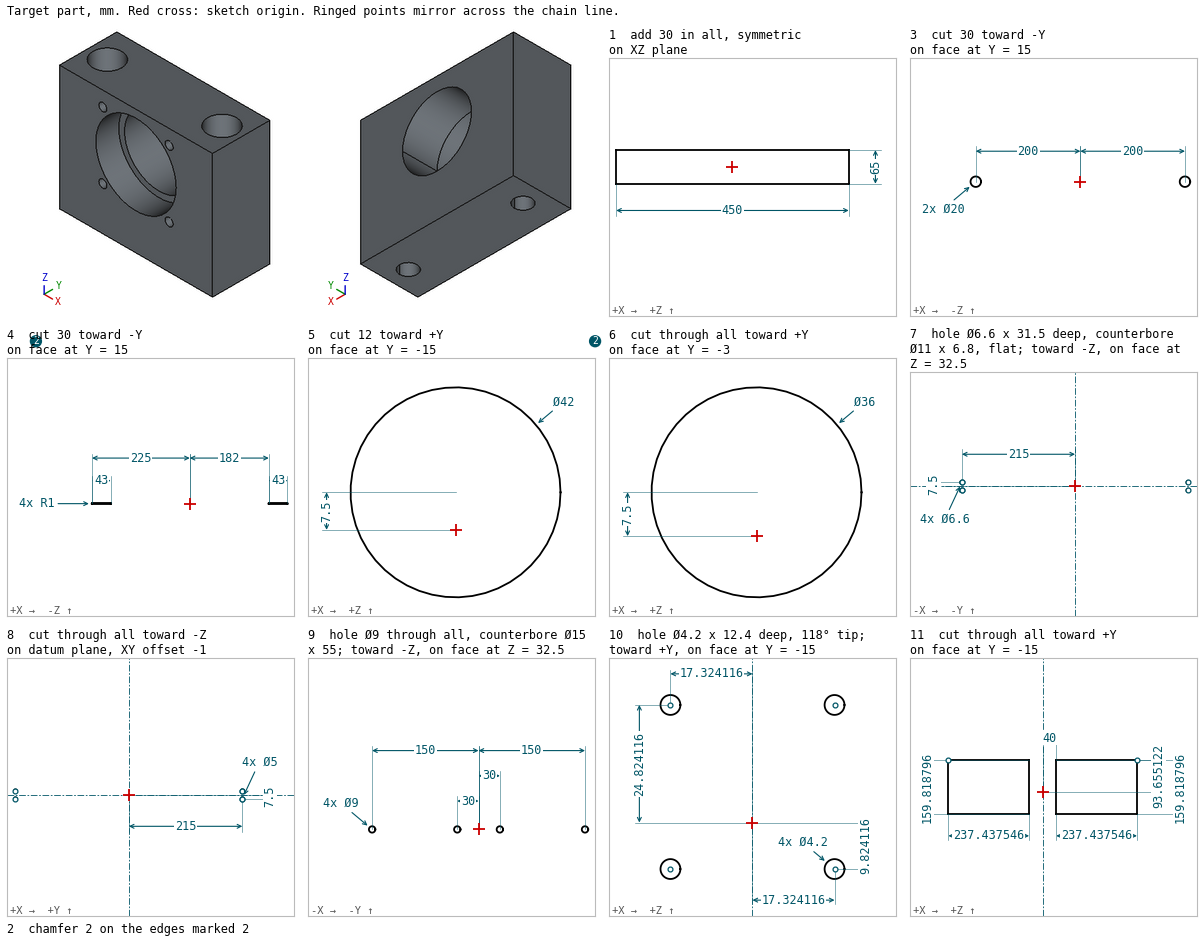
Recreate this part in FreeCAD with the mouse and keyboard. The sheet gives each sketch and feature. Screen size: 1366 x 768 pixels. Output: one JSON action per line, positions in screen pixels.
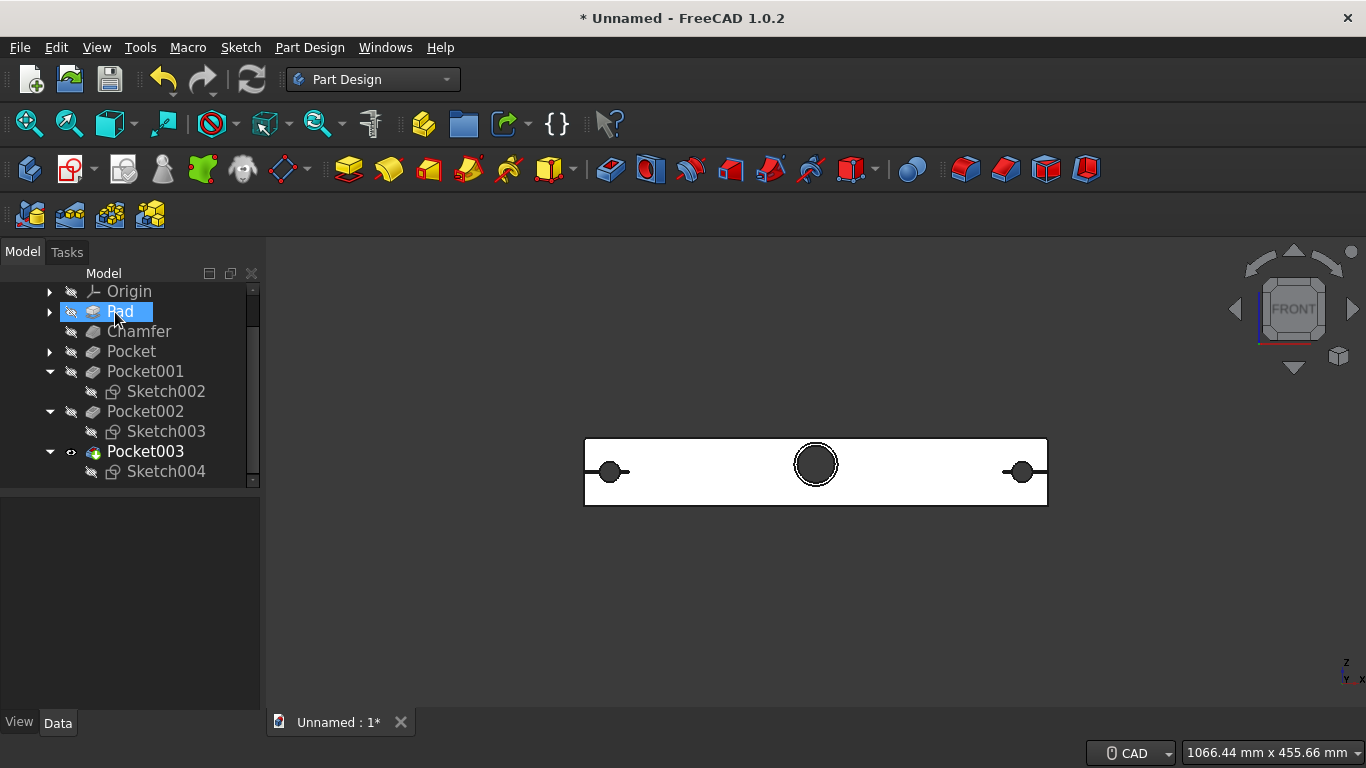
{"action": "key", "text": "0"}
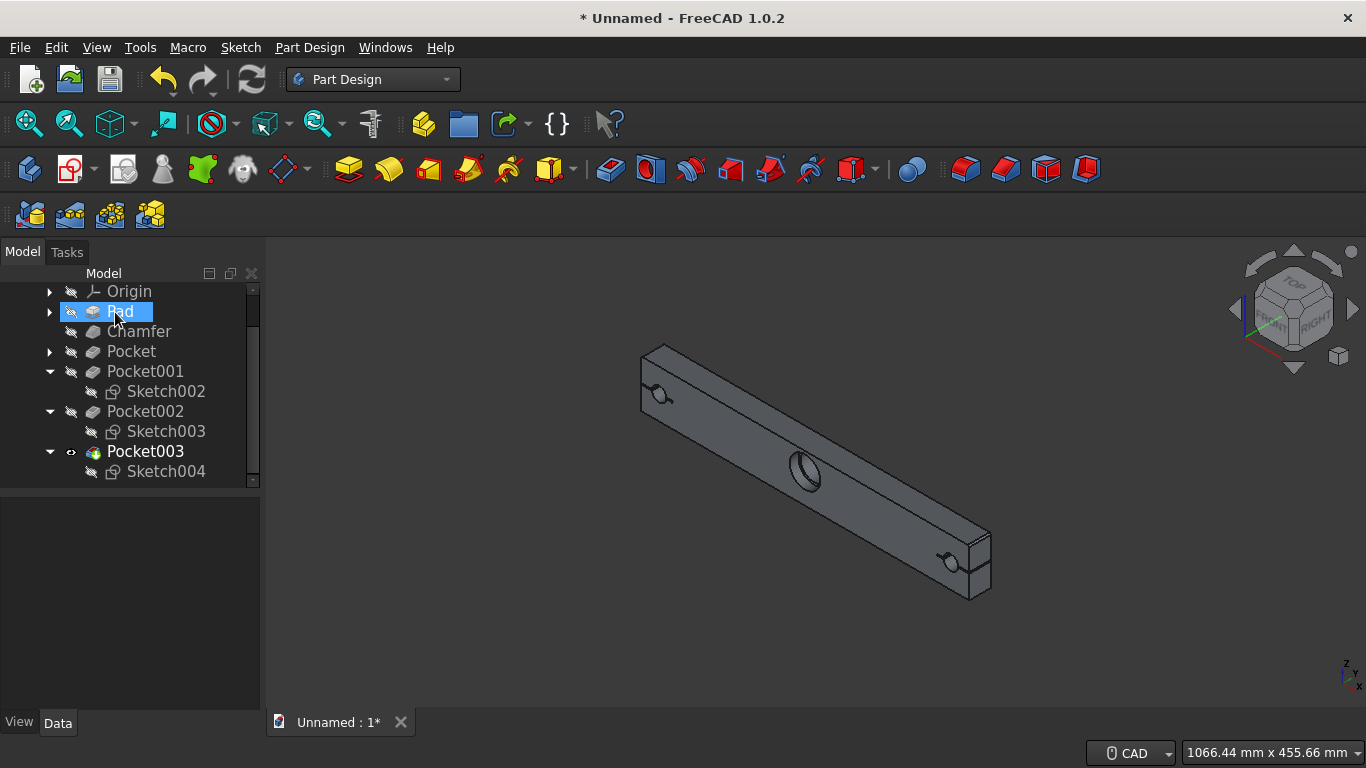
{"action": "left_click", "coordinate": [955, 524]}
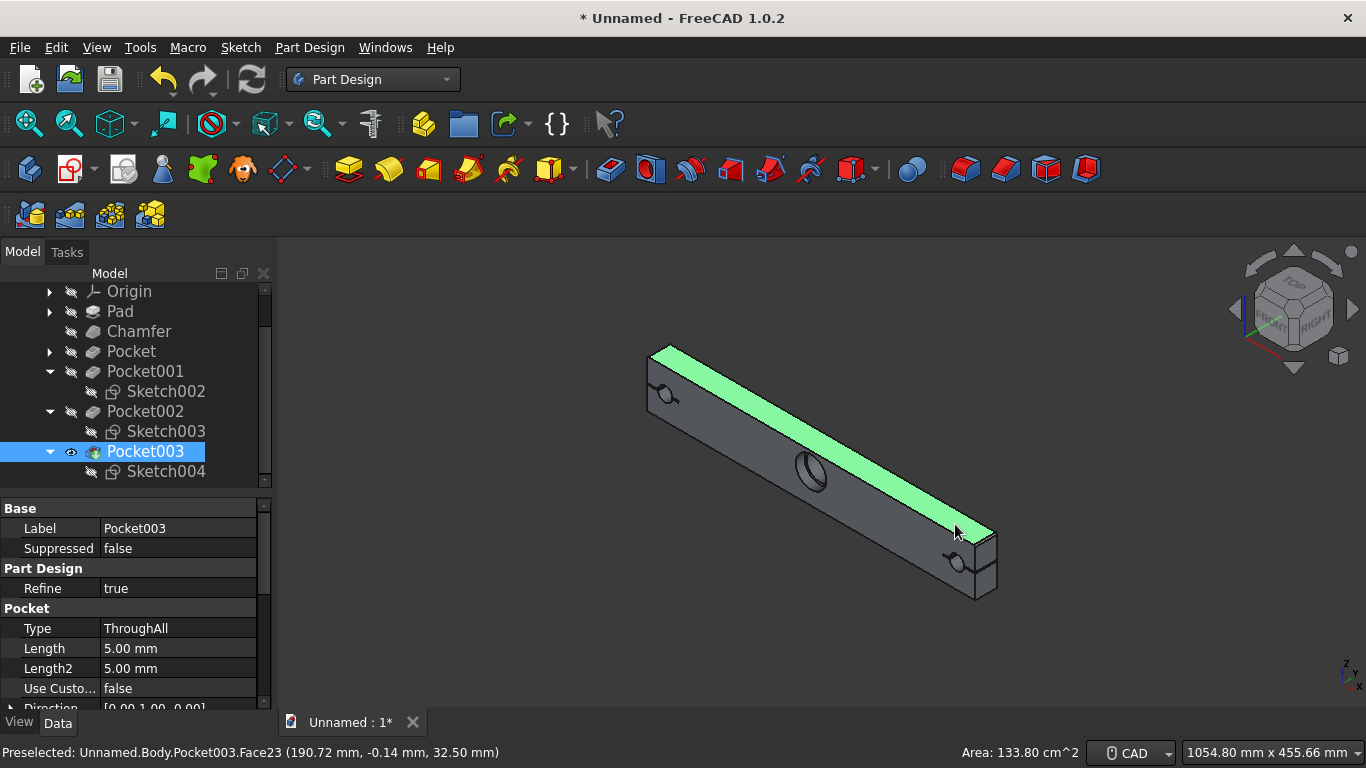
{"action": "left_click", "coordinate": [70, 170]}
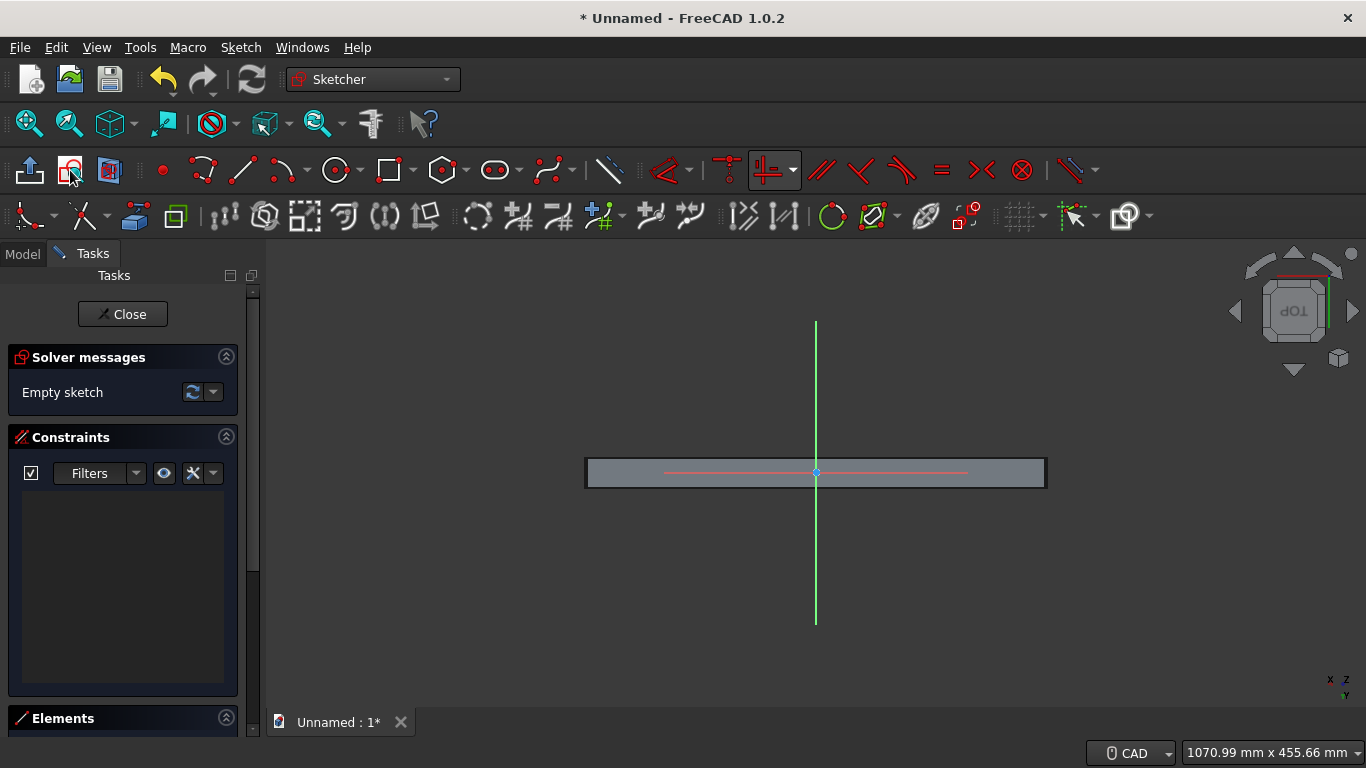
{"action": "scroll", "coordinate": [955, 473], "scroll_direction": "up", "scroll_amount": 2}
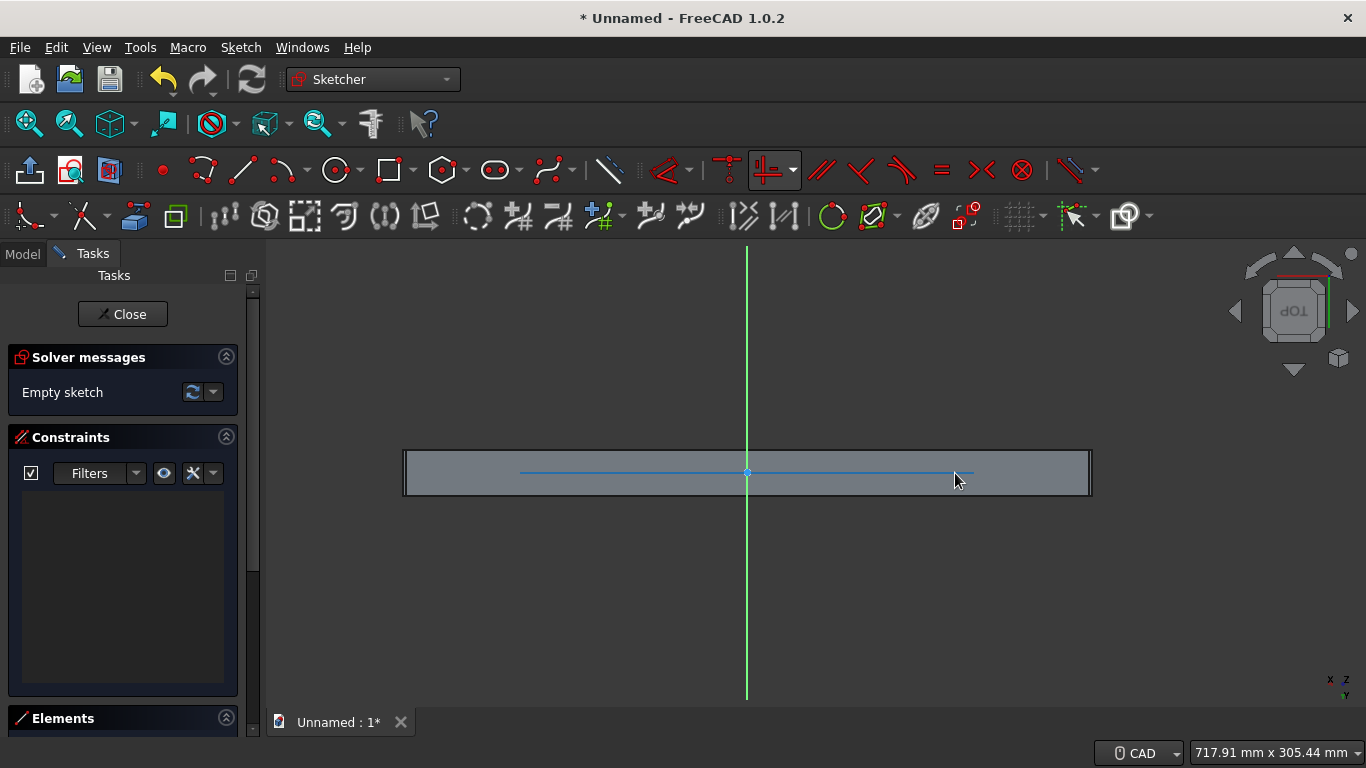
{"action": "key", "text": "g c"}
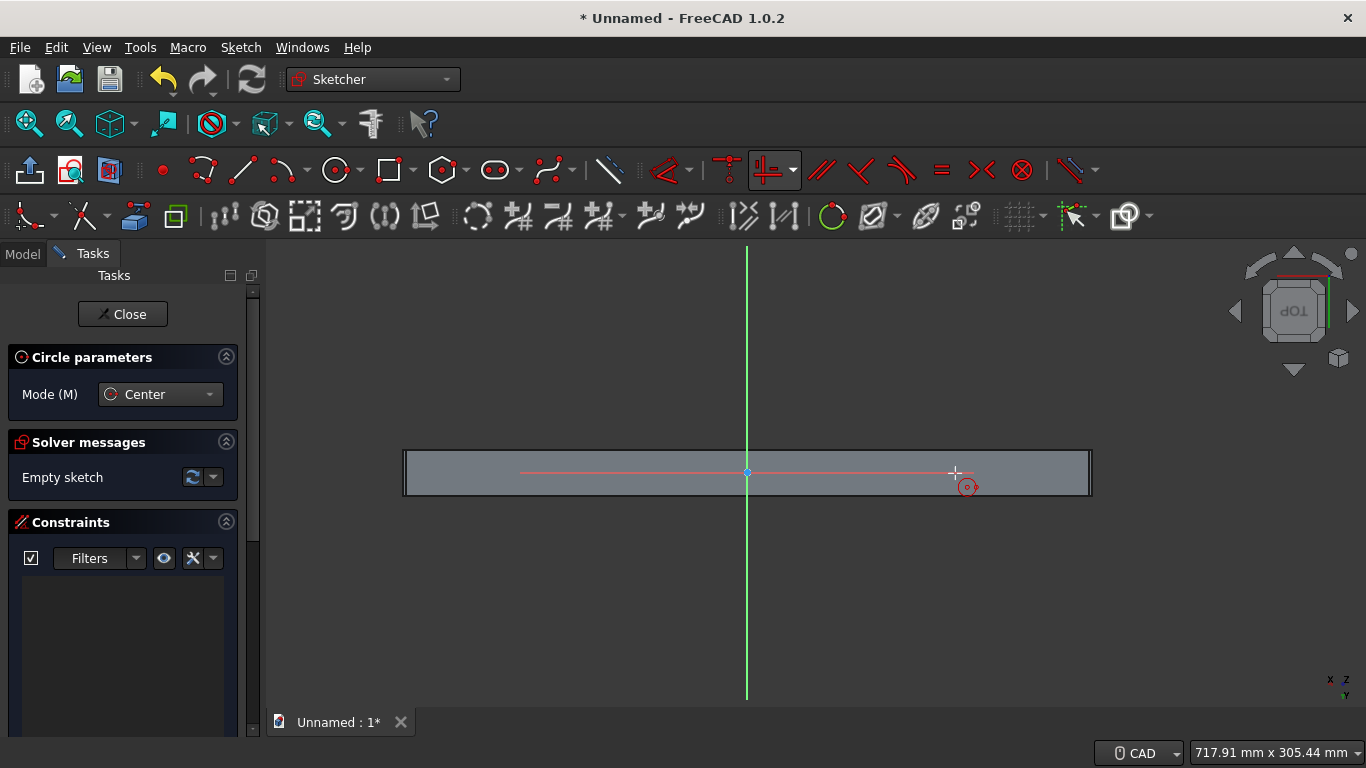
{"action": "scroll", "coordinate": [418, 461], "scroll_direction": "up", "scroll_amount": 8}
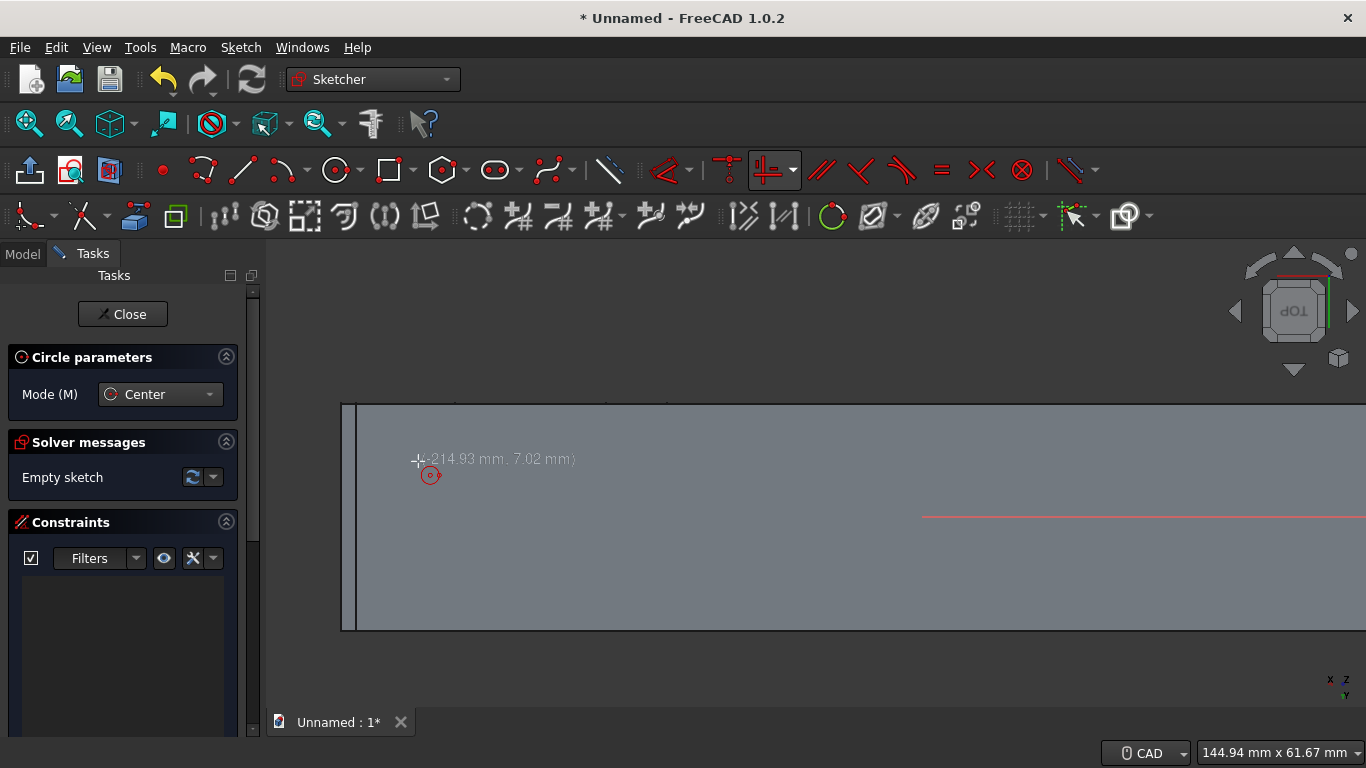
{"action": "scroll", "coordinate": [418, 462], "scroll_direction": "down", "scroll_amount": 8}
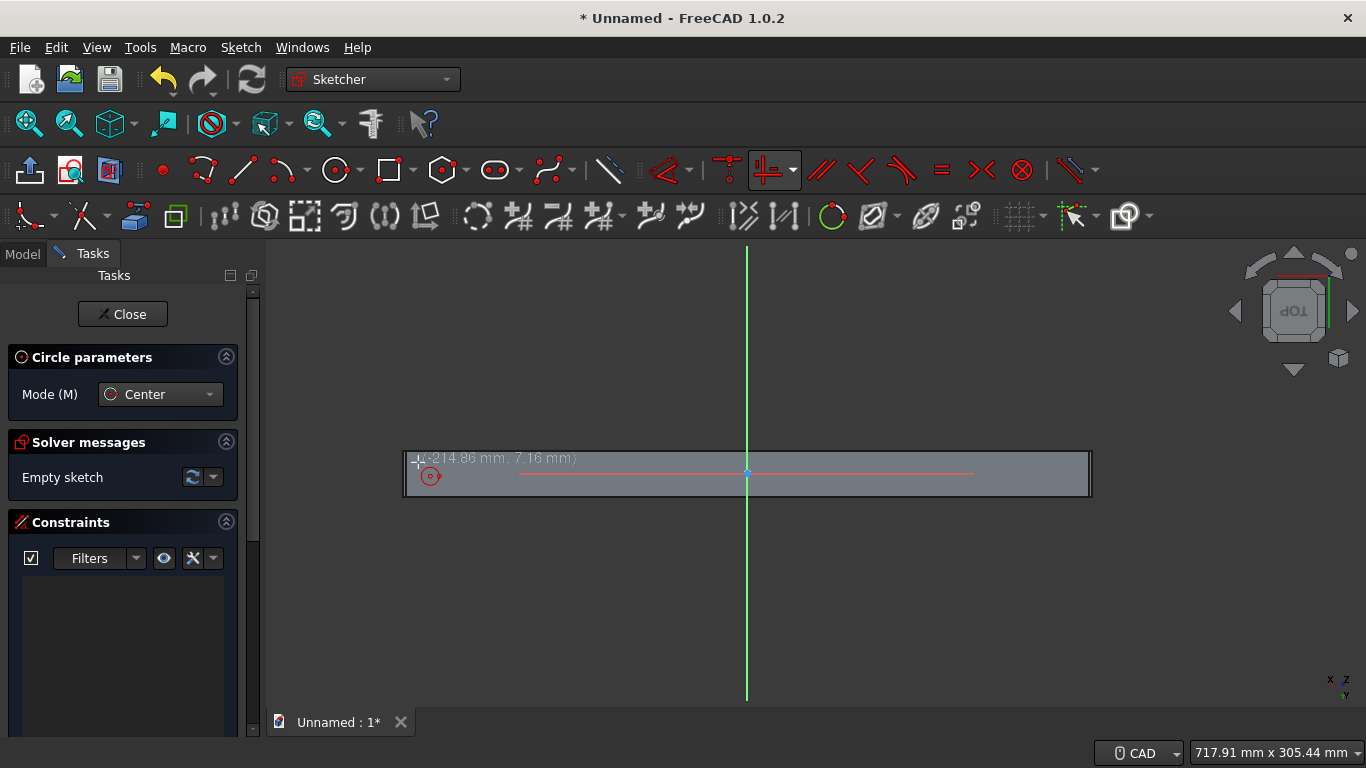
{"action": "scroll", "coordinate": [418, 462], "scroll_direction": "up", "scroll_amount": 2}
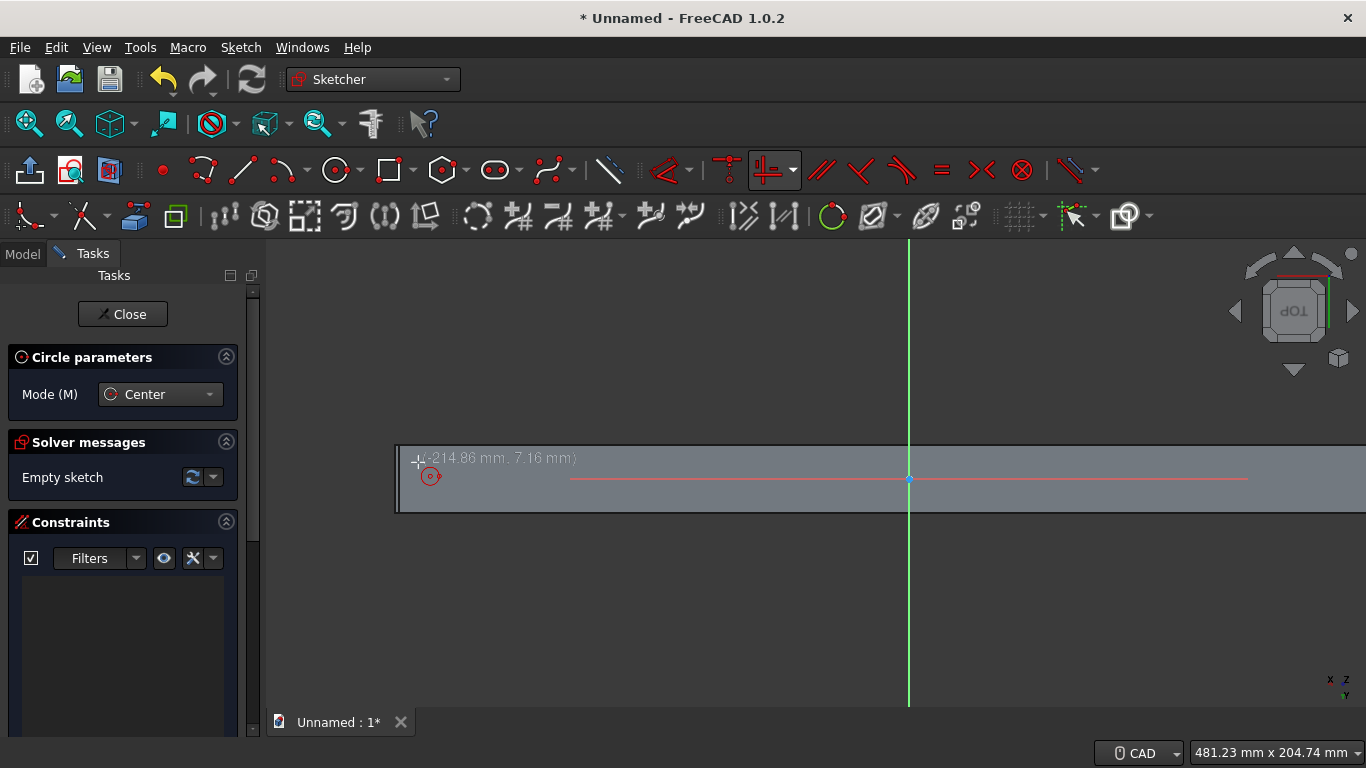
{"action": "left_click", "coordinate": [418, 462]}
{"action": "mouse_move", "coordinate": [423, 457]}